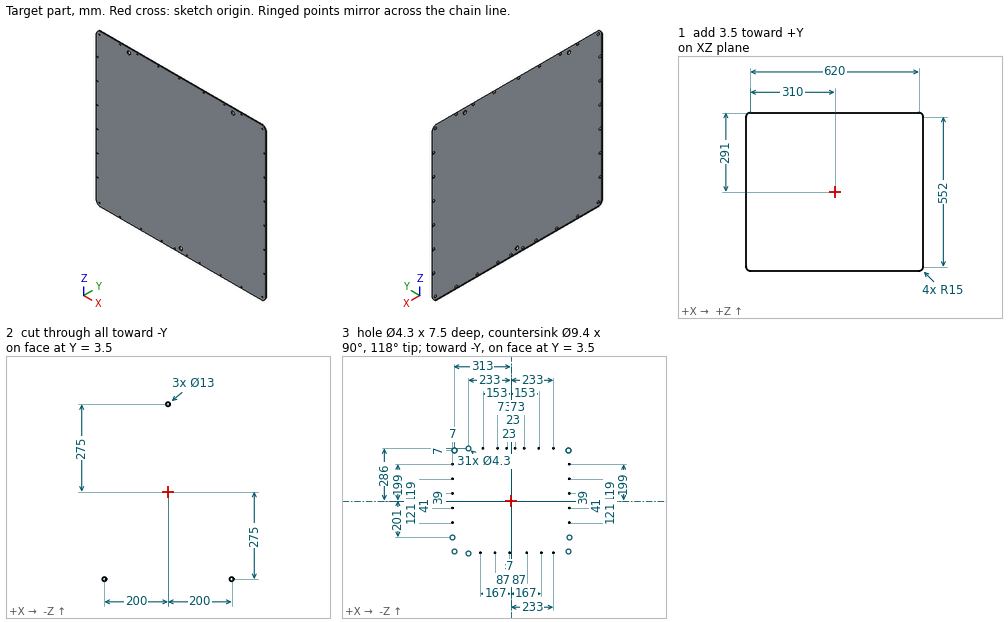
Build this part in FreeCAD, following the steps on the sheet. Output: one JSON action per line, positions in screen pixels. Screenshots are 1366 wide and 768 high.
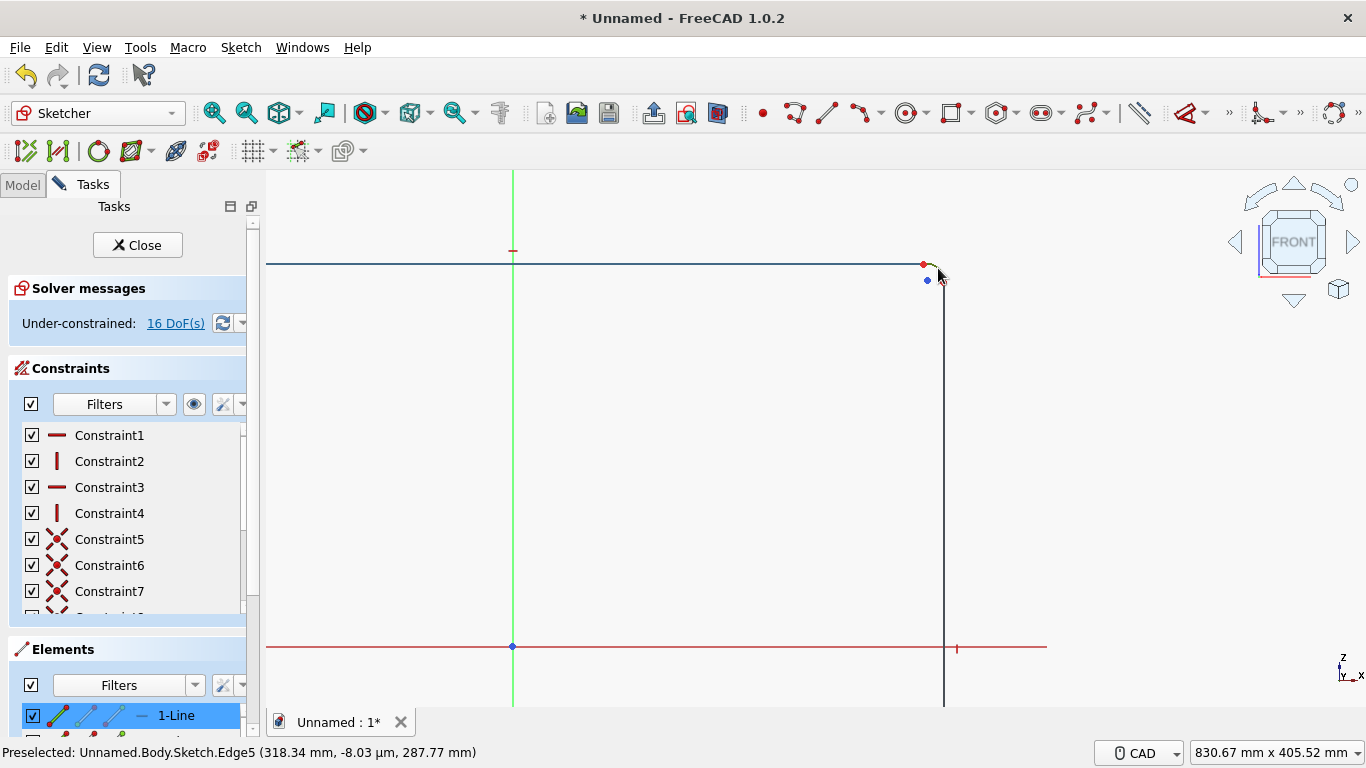
{"action": "key", "text": "t"}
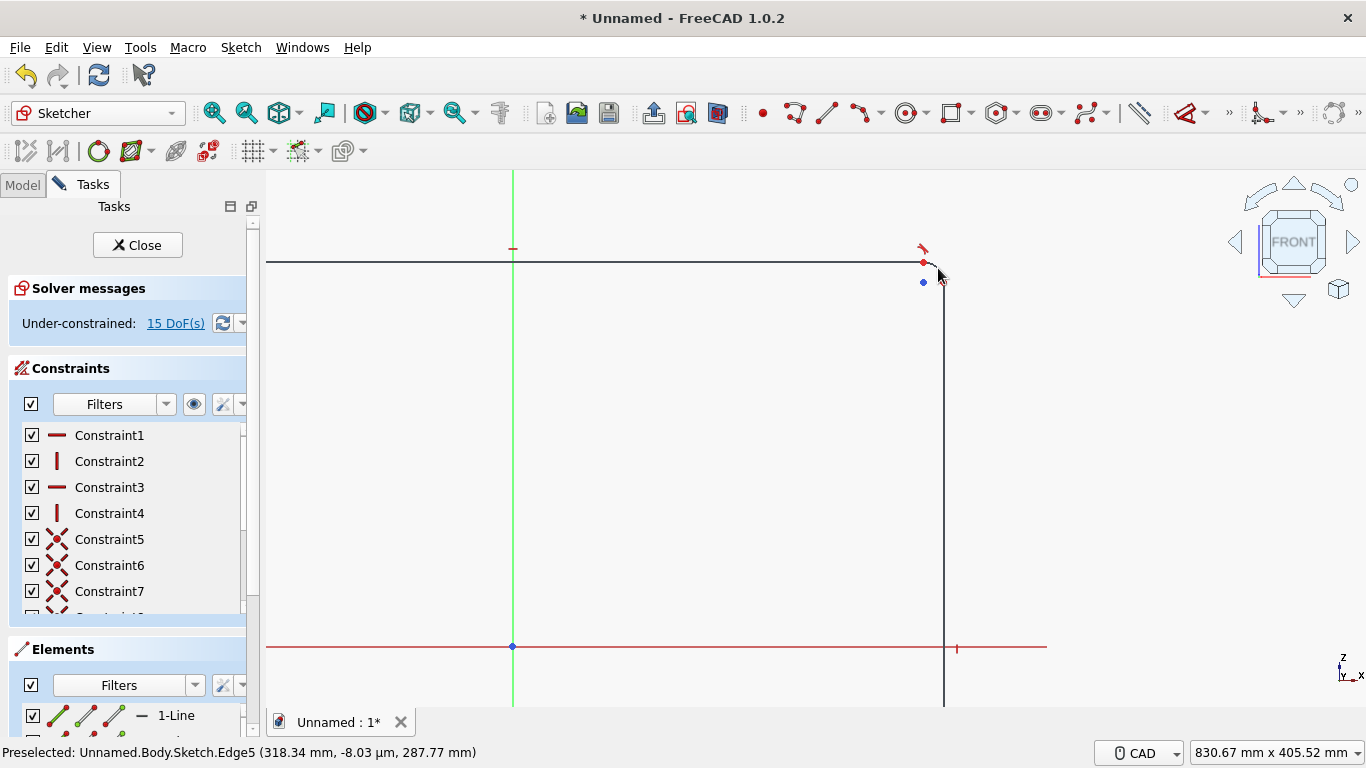
{"action": "left_click", "coordinate": [349, 262]}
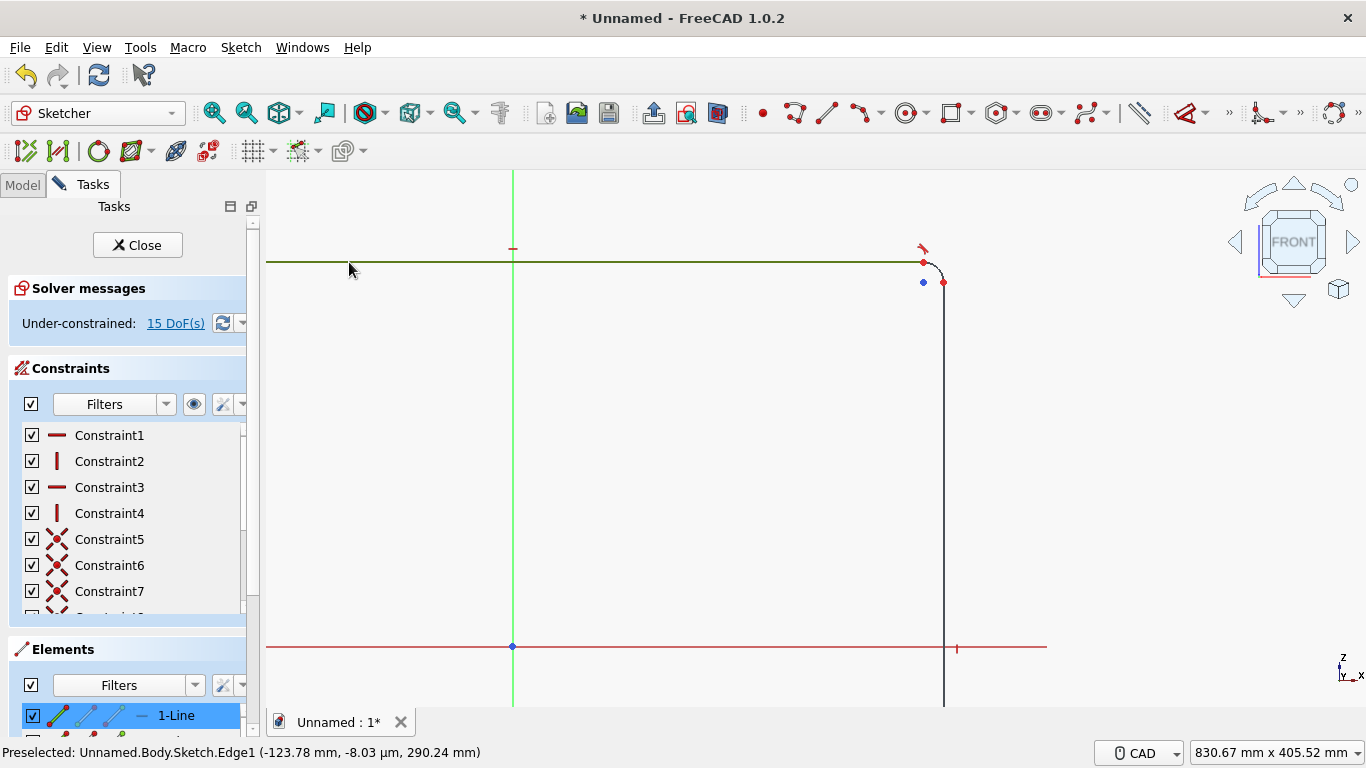
{"action": "scroll", "coordinate": [939, 269], "scroll_direction": "down", "scroll_amount": 4}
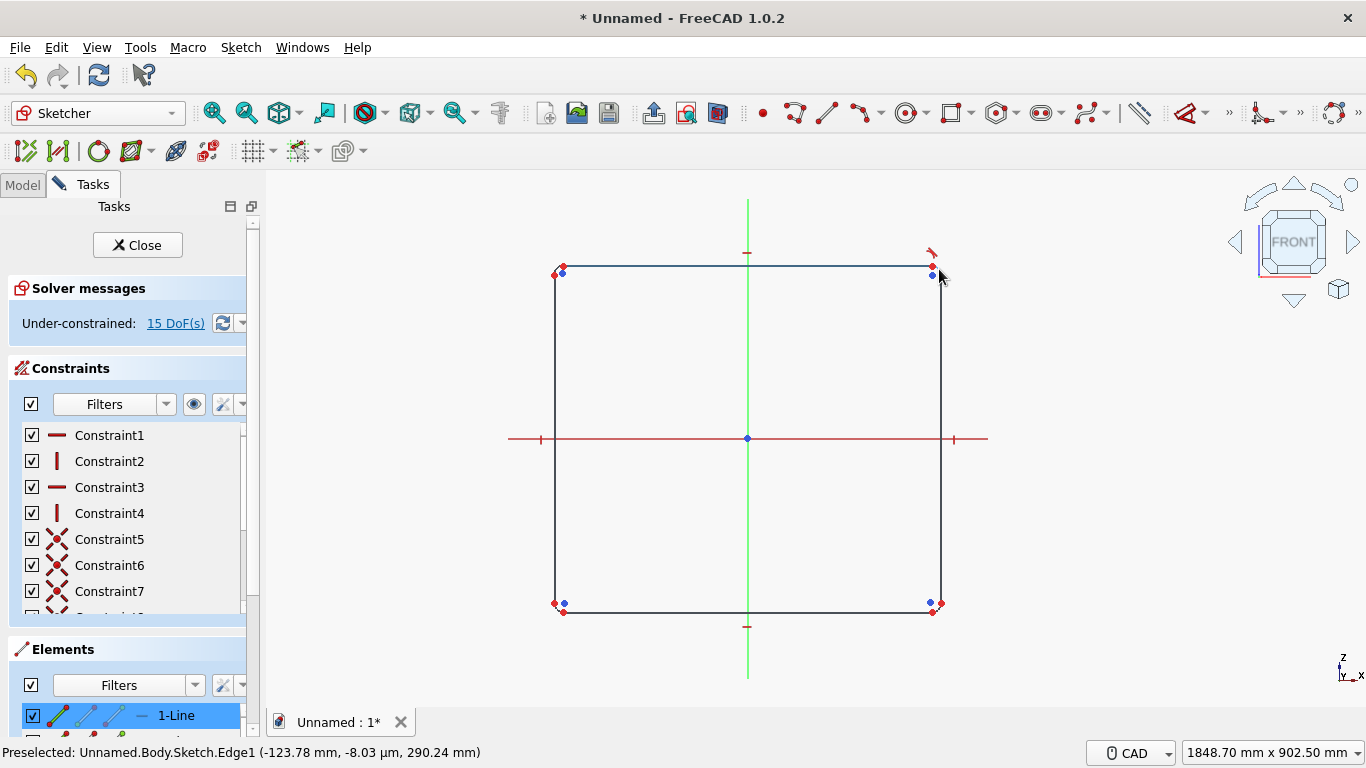
{"action": "scroll", "coordinate": [559, 267], "scroll_direction": "up", "scroll_amount": 6}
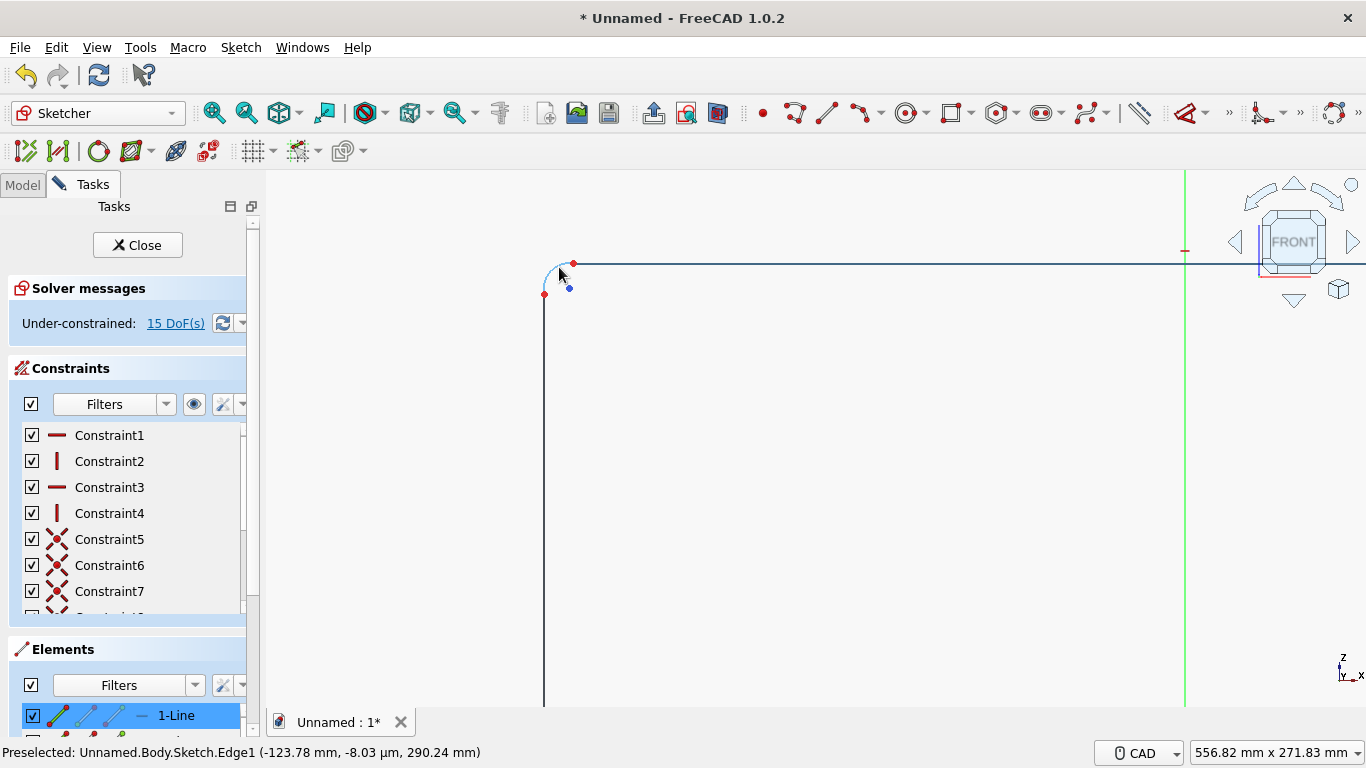
{"action": "left_click", "coordinate": [559, 265]}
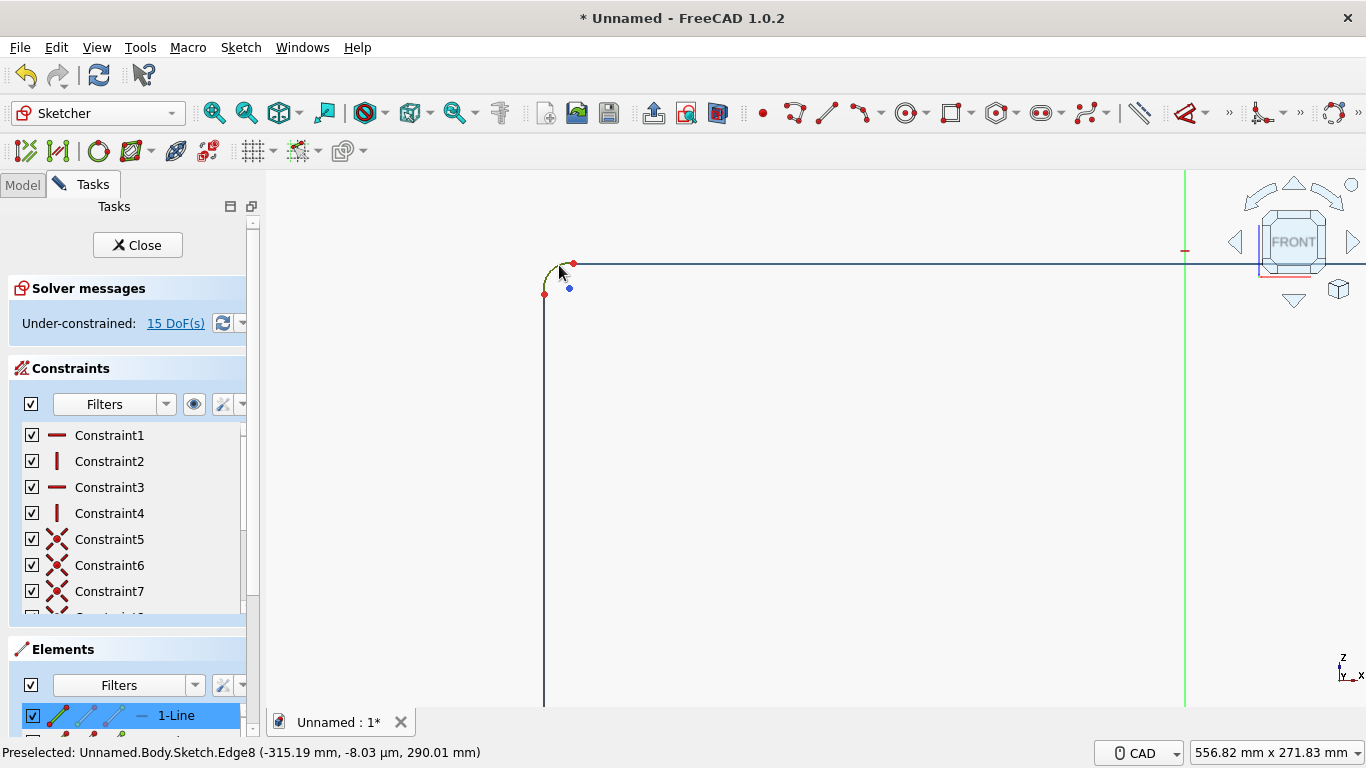
{"action": "key", "text": "t"}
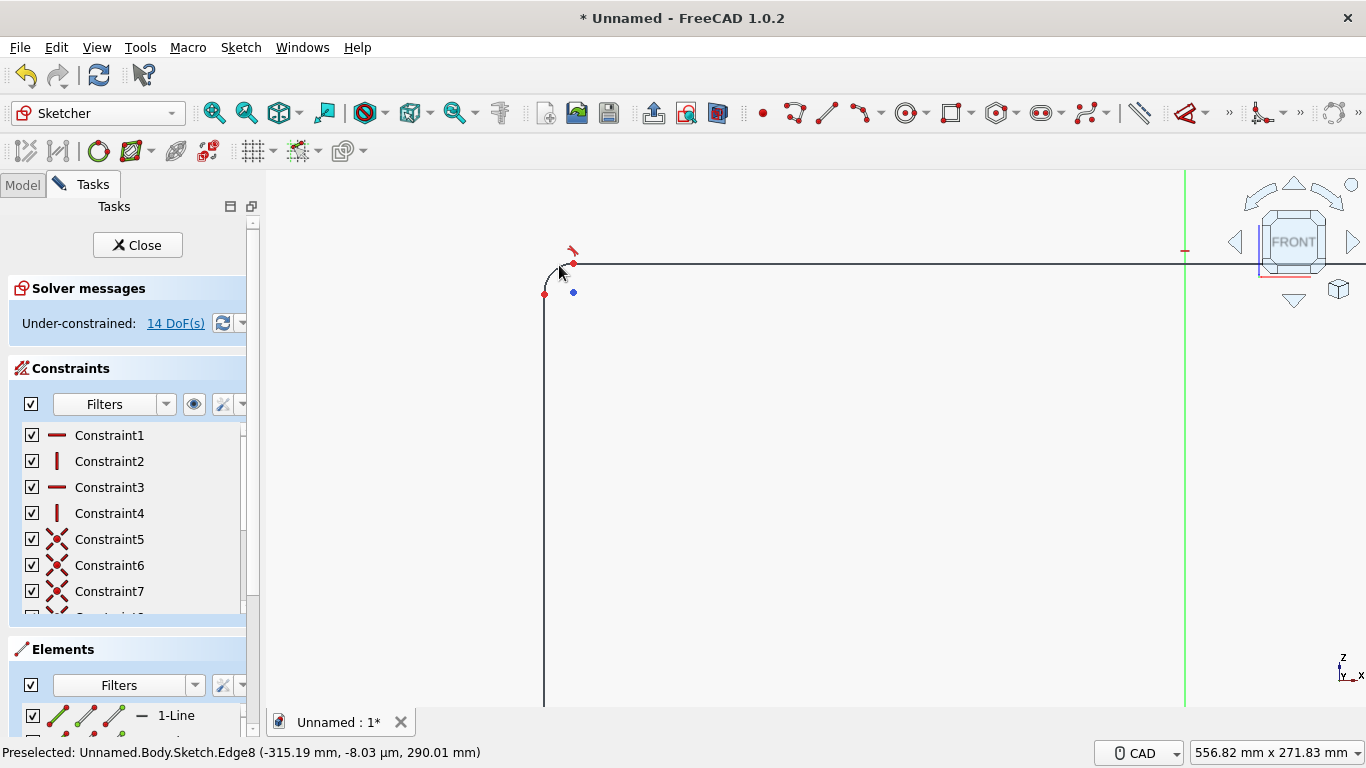
{"action": "scroll", "coordinate": [559, 267], "scroll_direction": "down", "scroll_amount": 6}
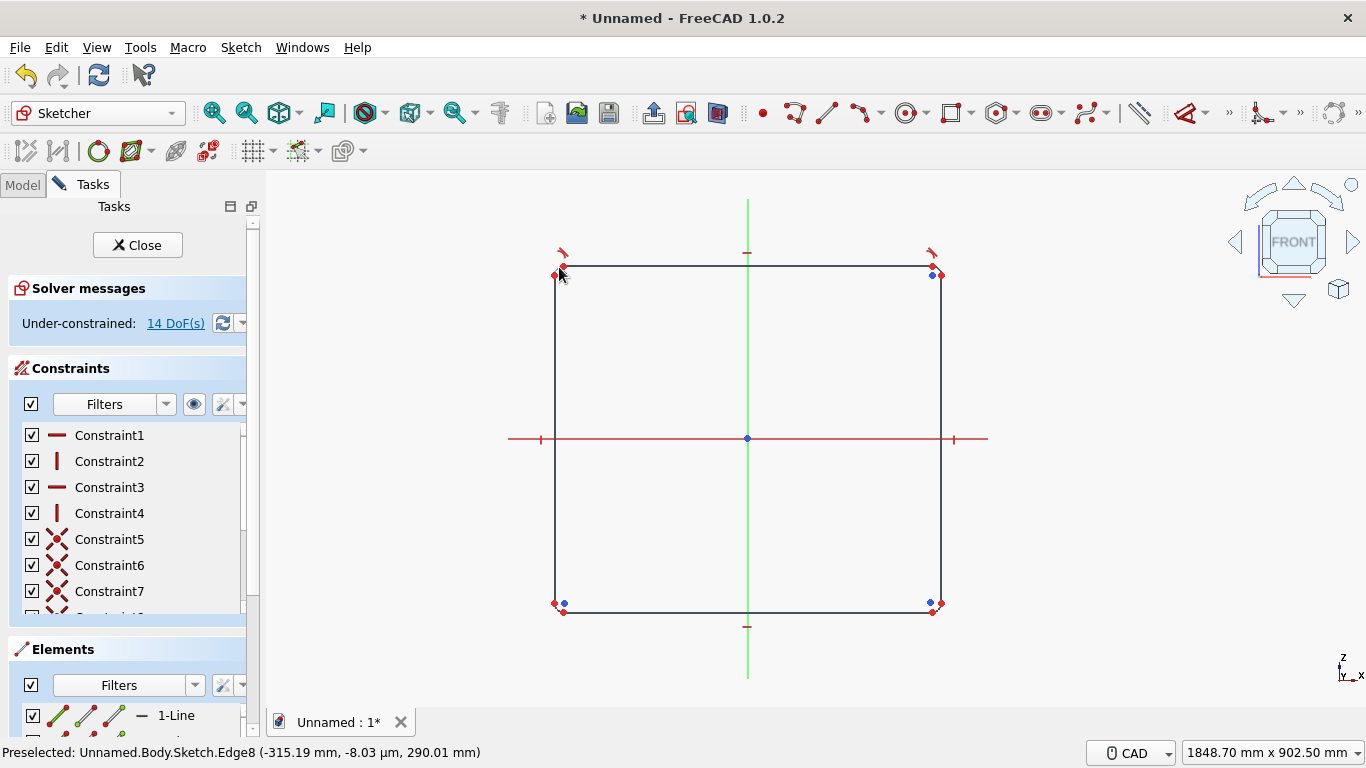
{"action": "left_click", "coordinate": [941, 374]}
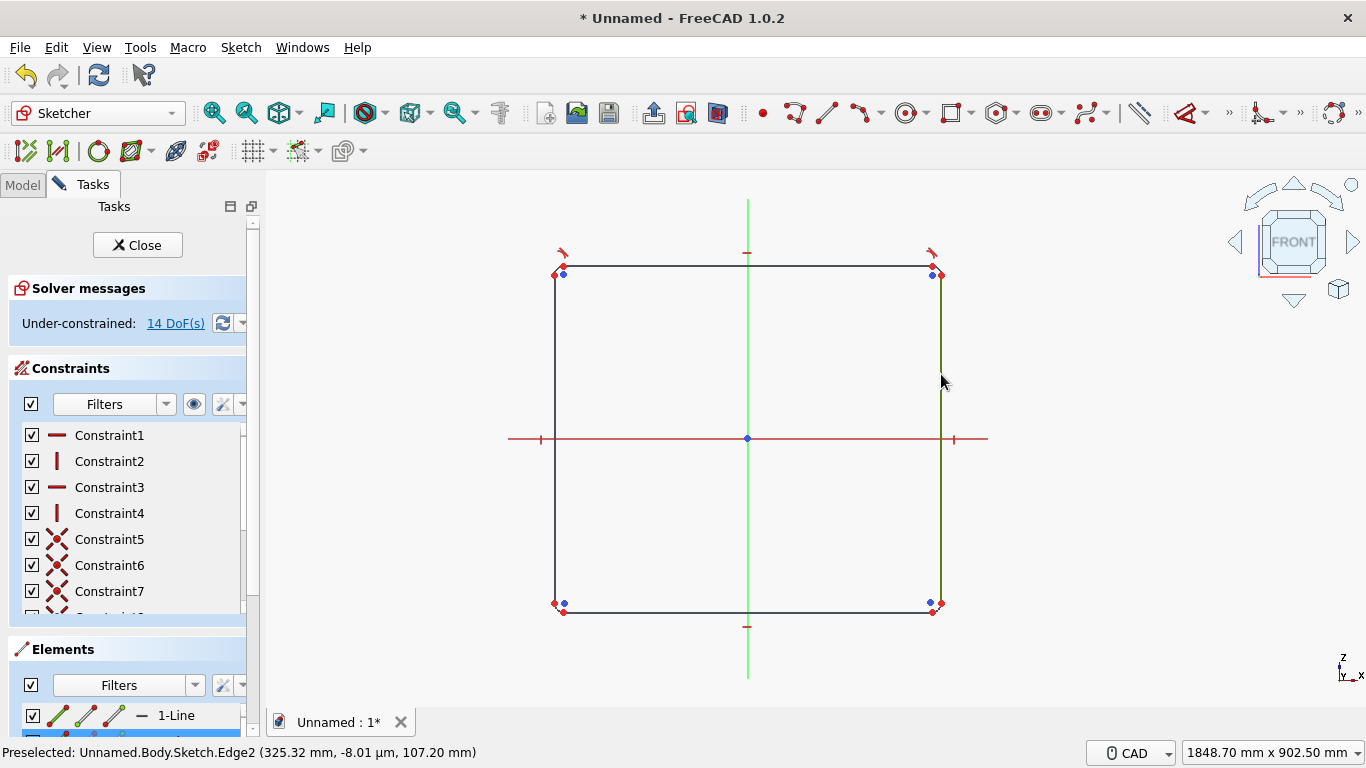
{"action": "scroll", "coordinate": [939, 269], "scroll_direction": "up", "scroll_amount": 4}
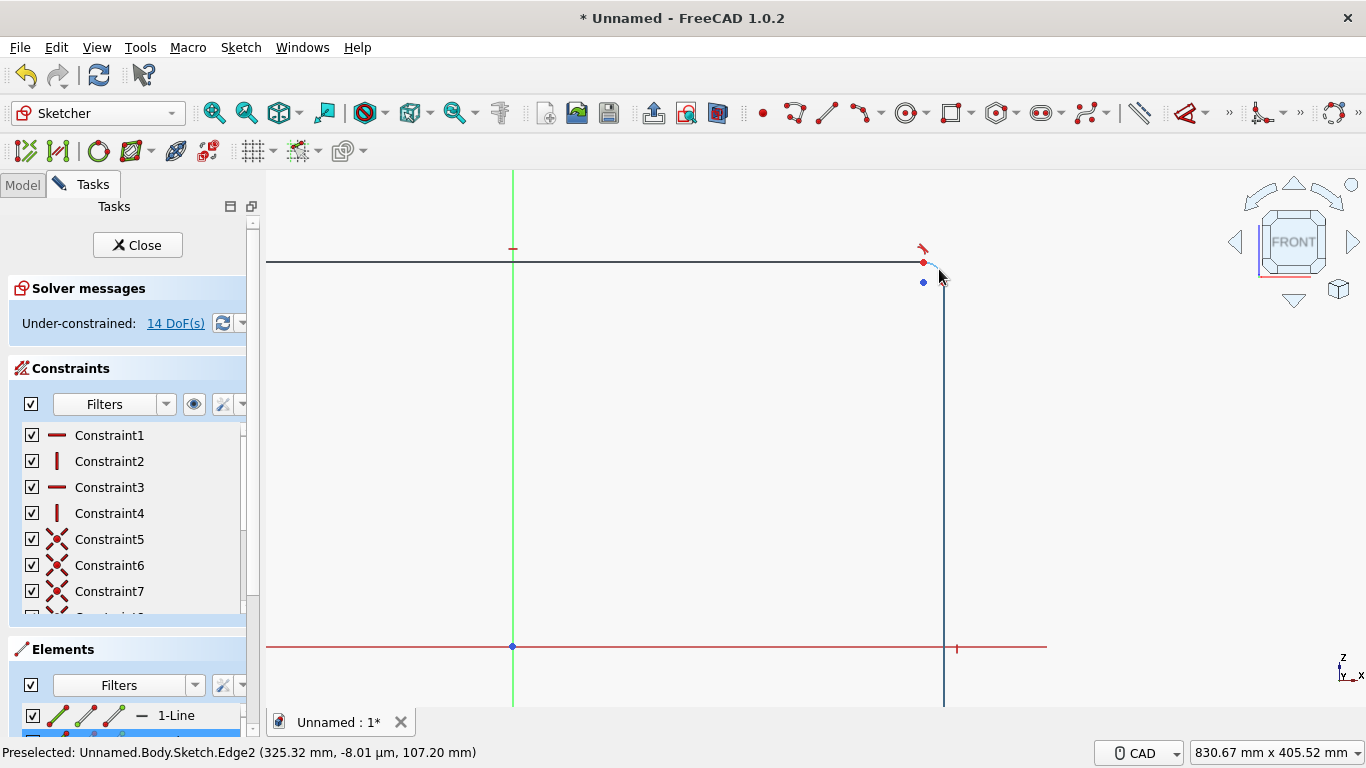
{"action": "left_click", "coordinate": [938, 268]}